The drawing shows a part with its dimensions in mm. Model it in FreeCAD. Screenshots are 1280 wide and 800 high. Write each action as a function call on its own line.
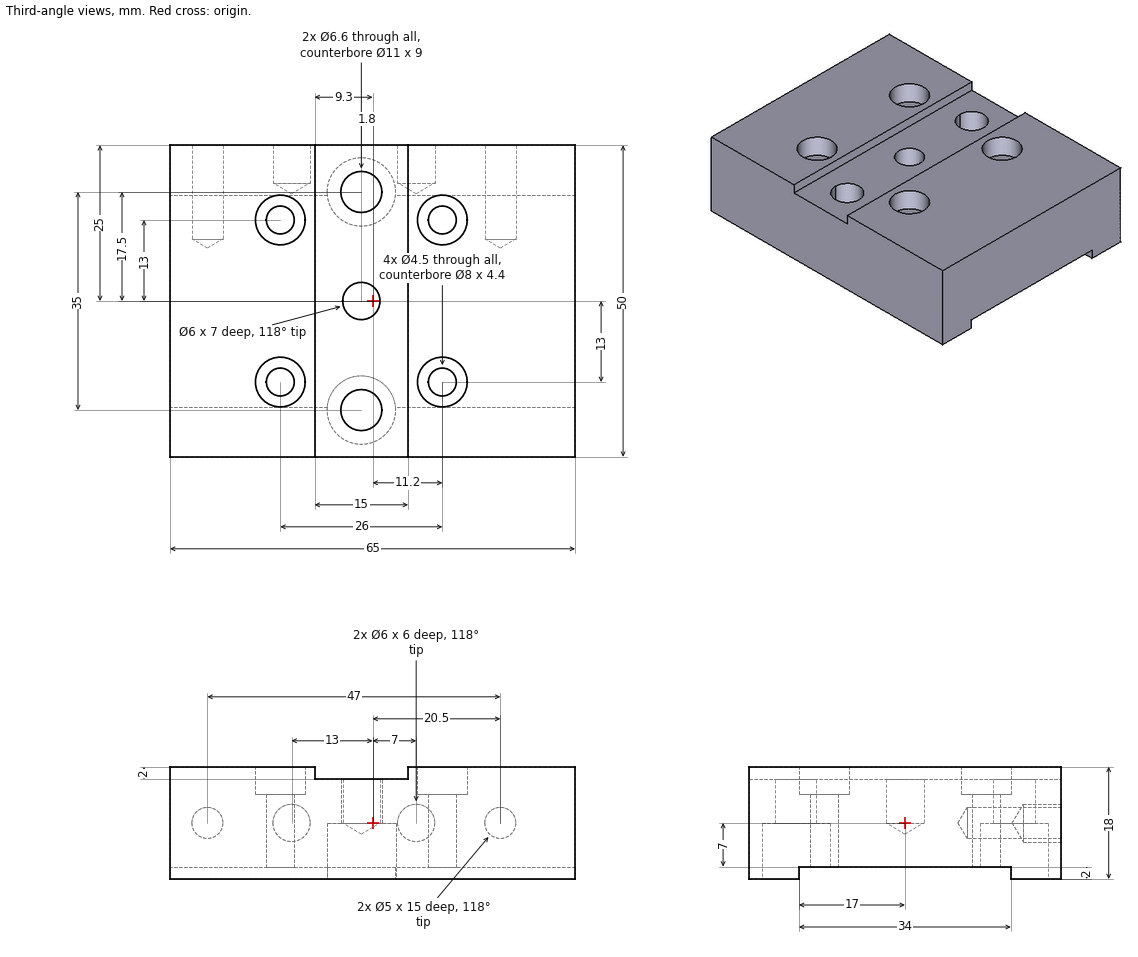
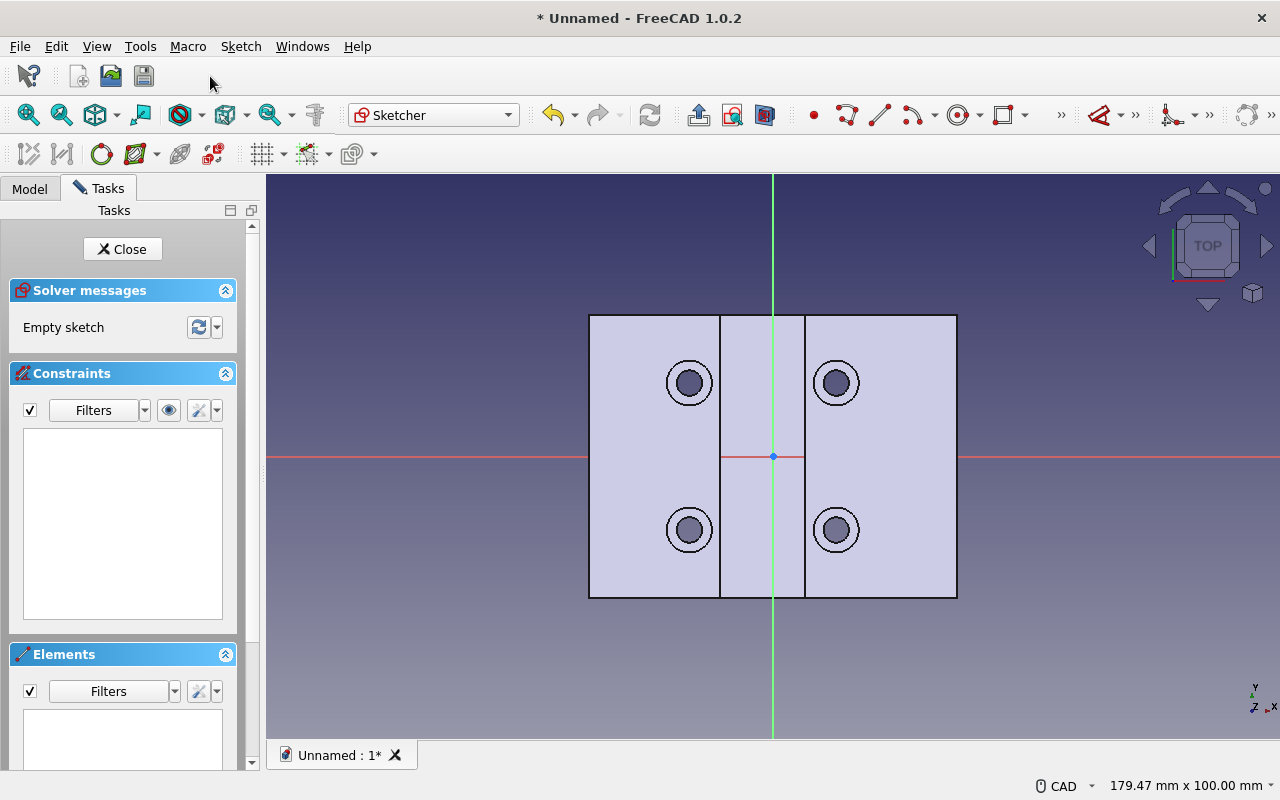
key(q)
key(s)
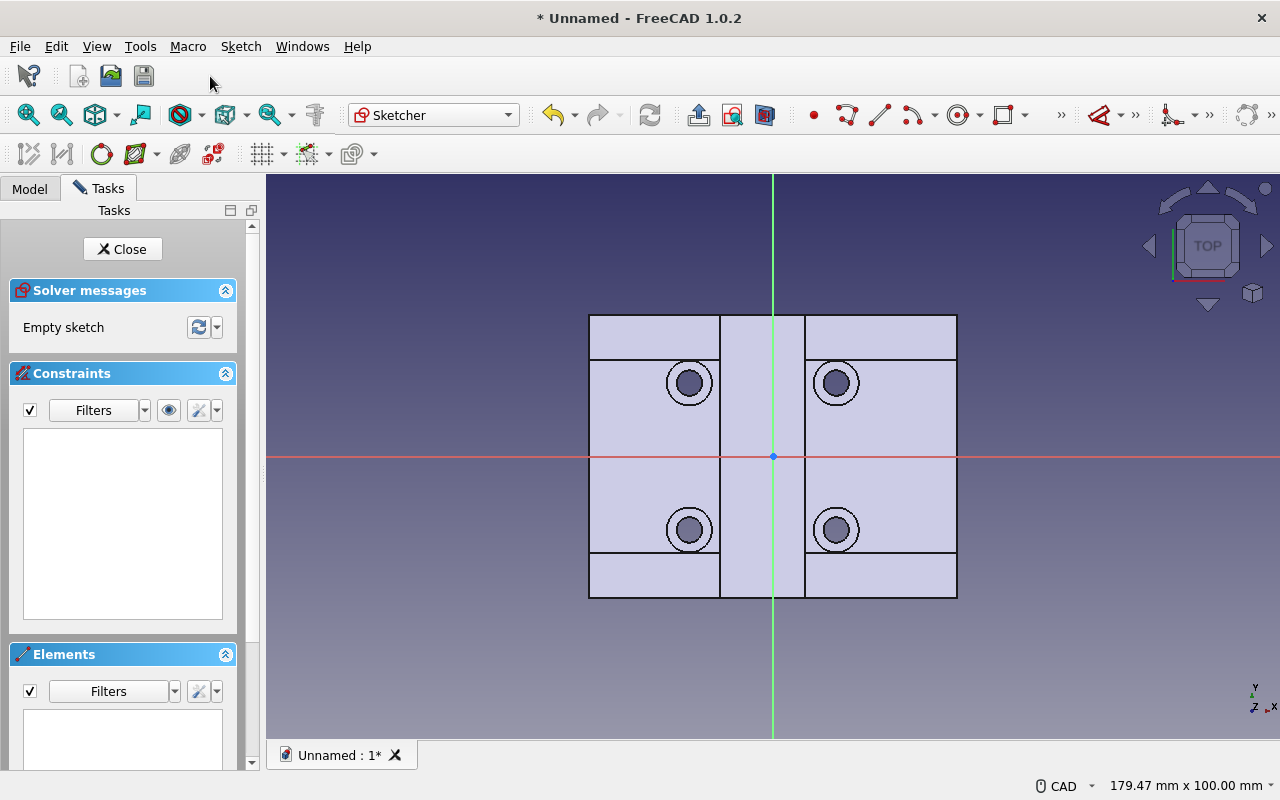
scroll(769, 456, up, 12)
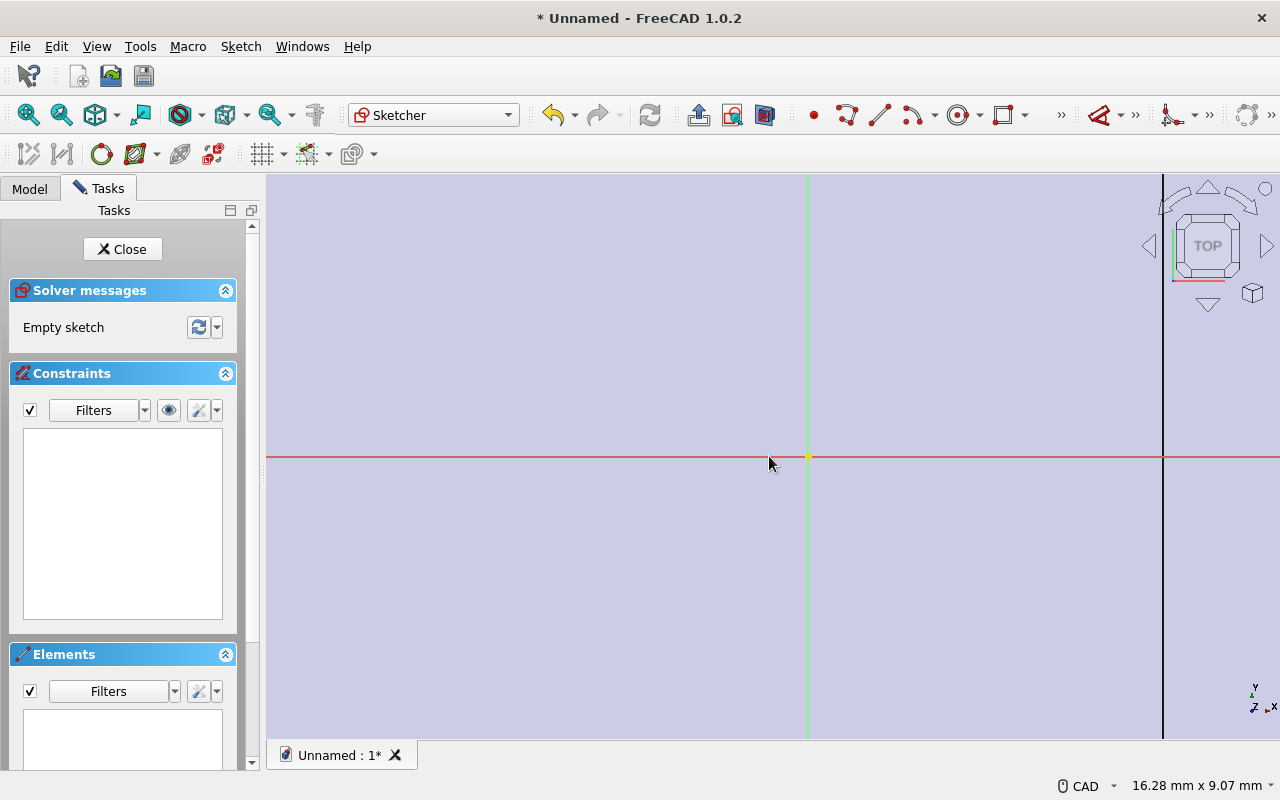
click(958, 116)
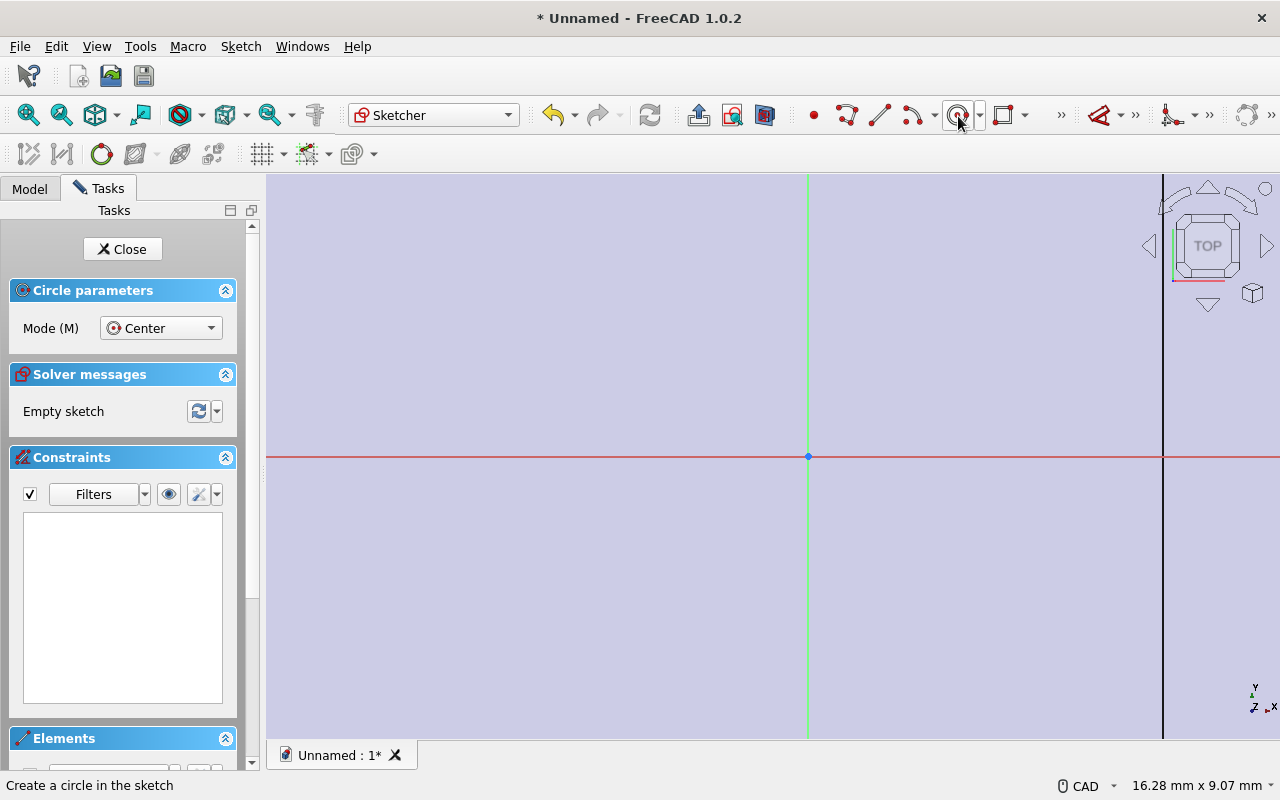
click(696, 456)
move(828, 324)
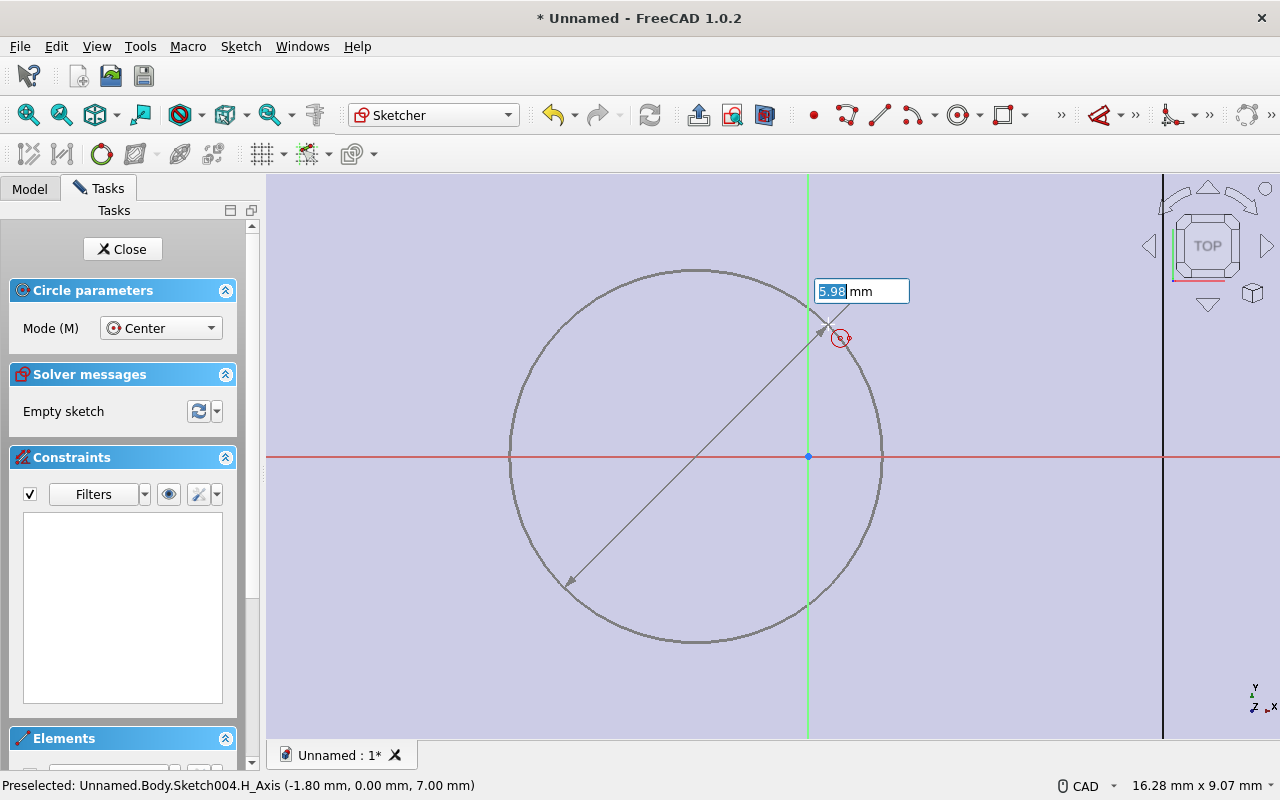
text(6)
key(Return)
key(Escape)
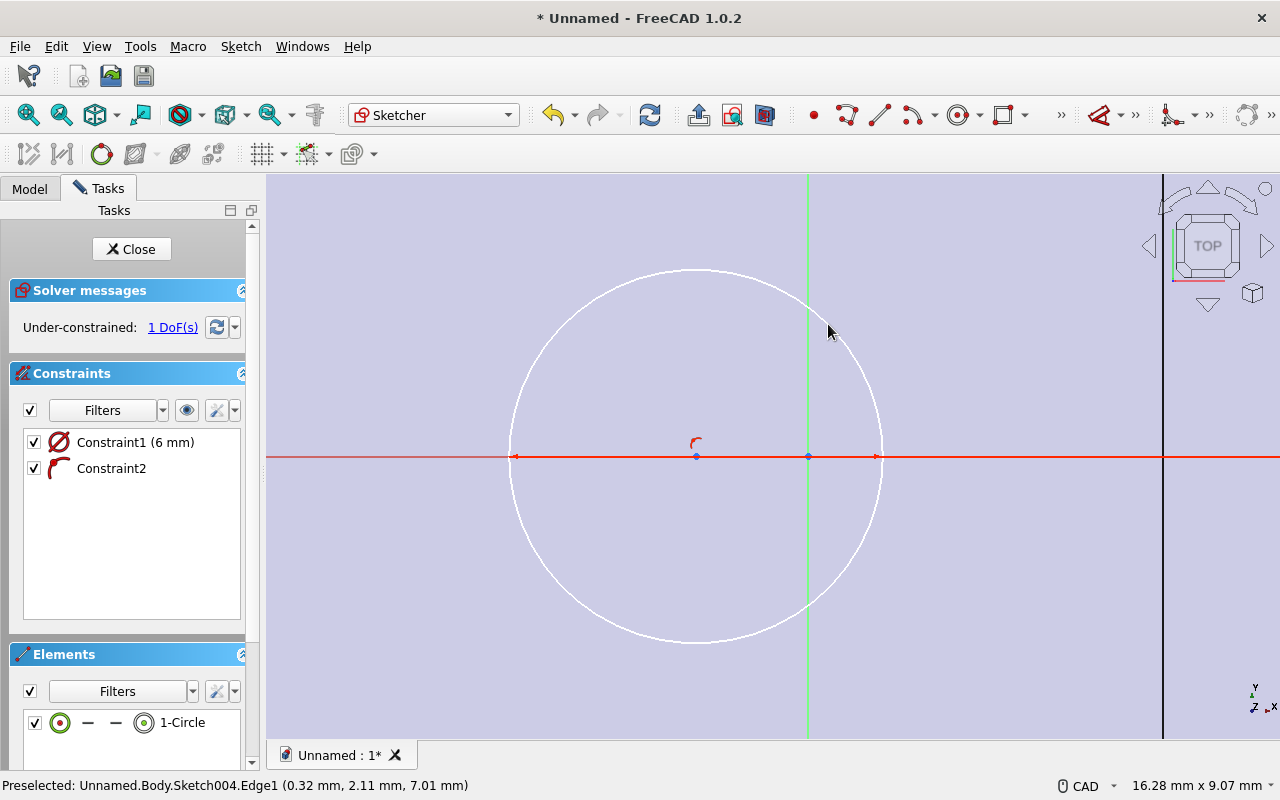
key(d)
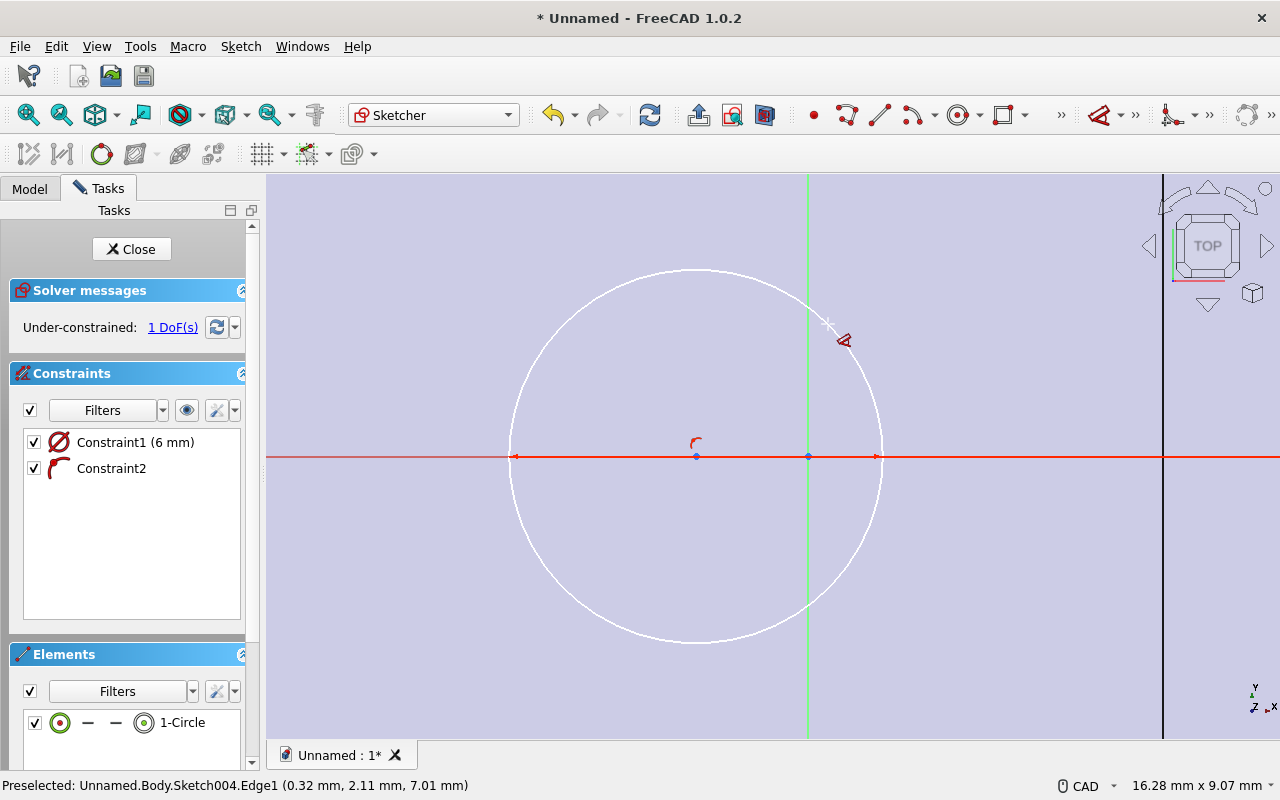
click(696, 456)
click(752, 490)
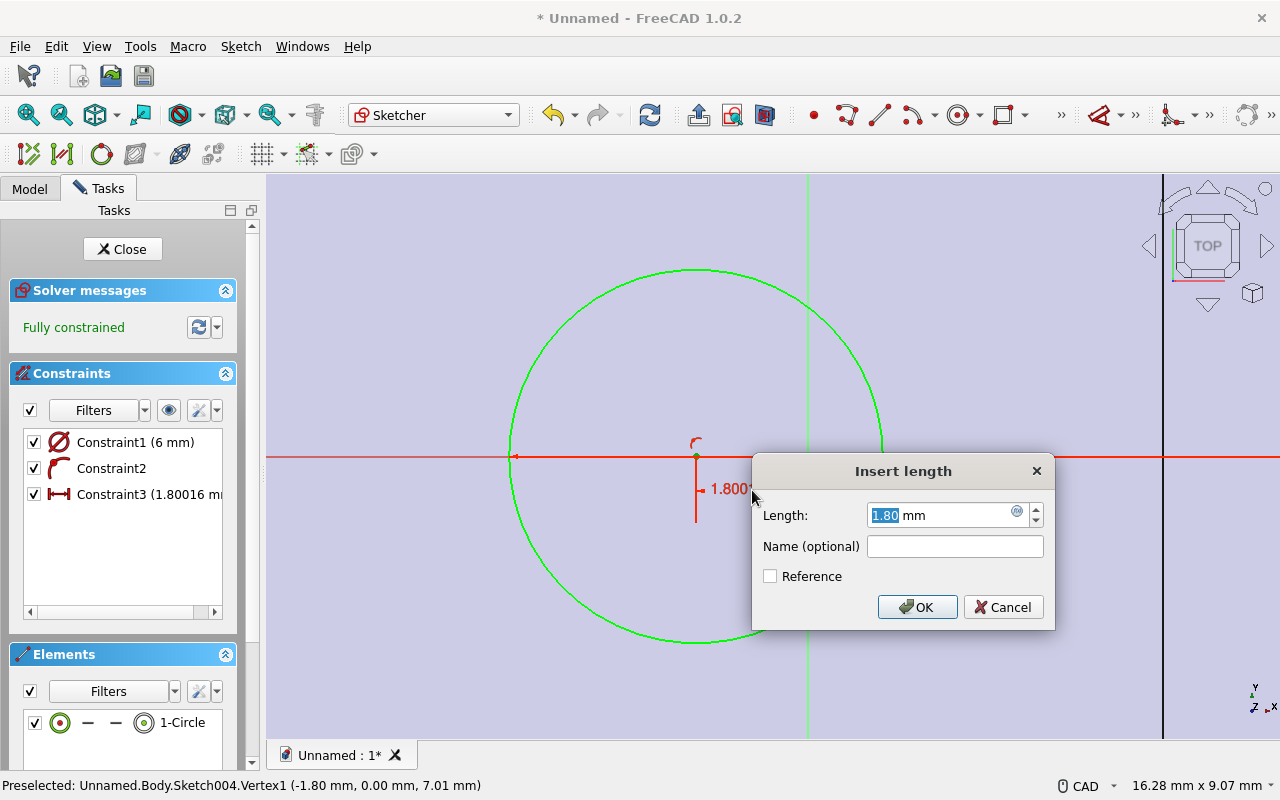
text(1.8)
key(Return)
key(Escape)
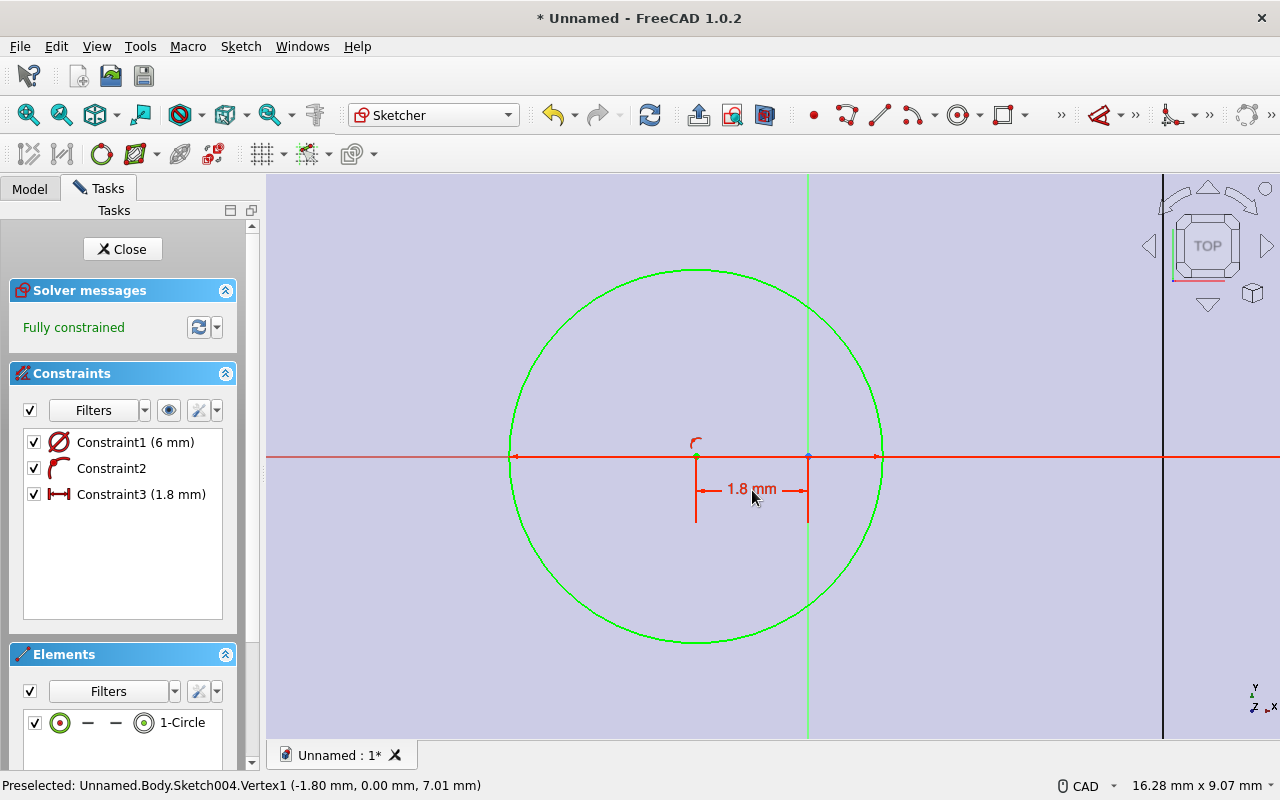
click(123, 249)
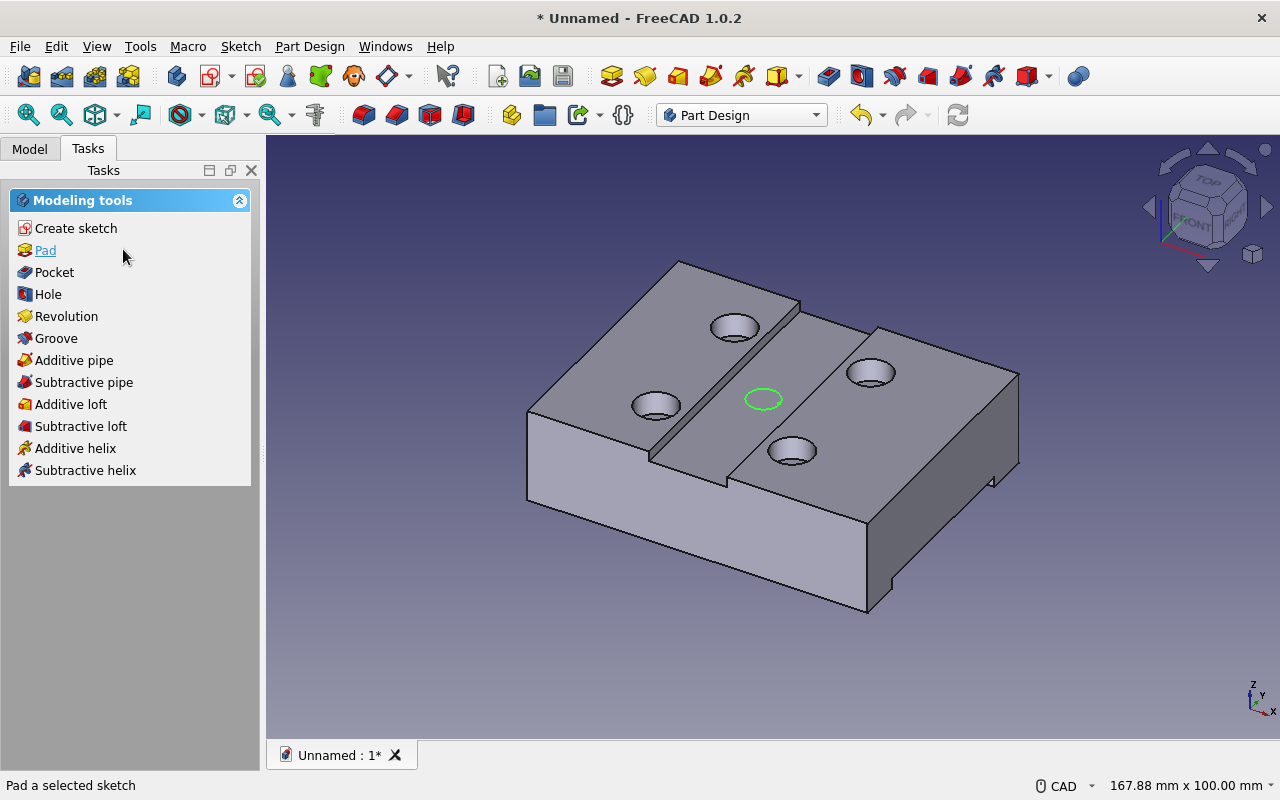
click(862, 76)